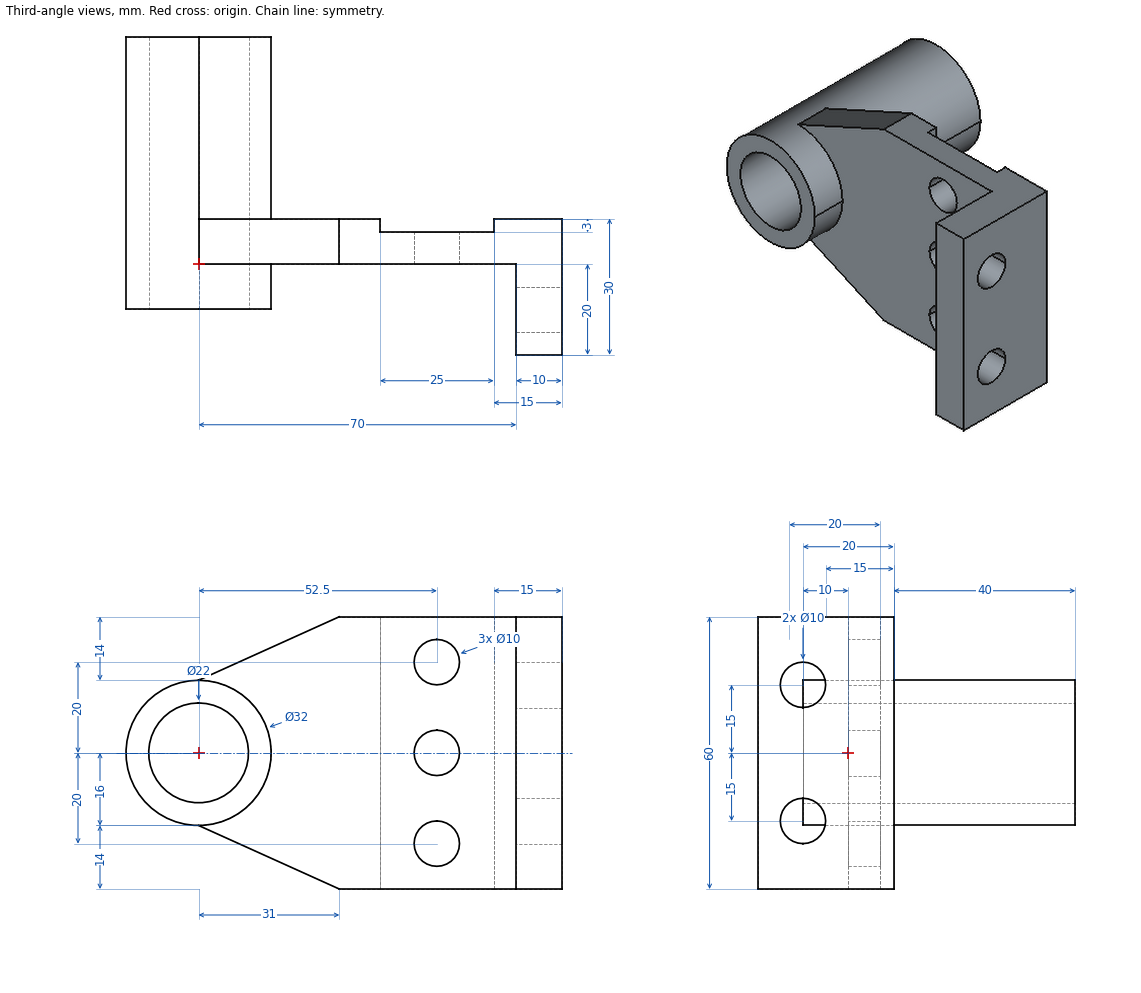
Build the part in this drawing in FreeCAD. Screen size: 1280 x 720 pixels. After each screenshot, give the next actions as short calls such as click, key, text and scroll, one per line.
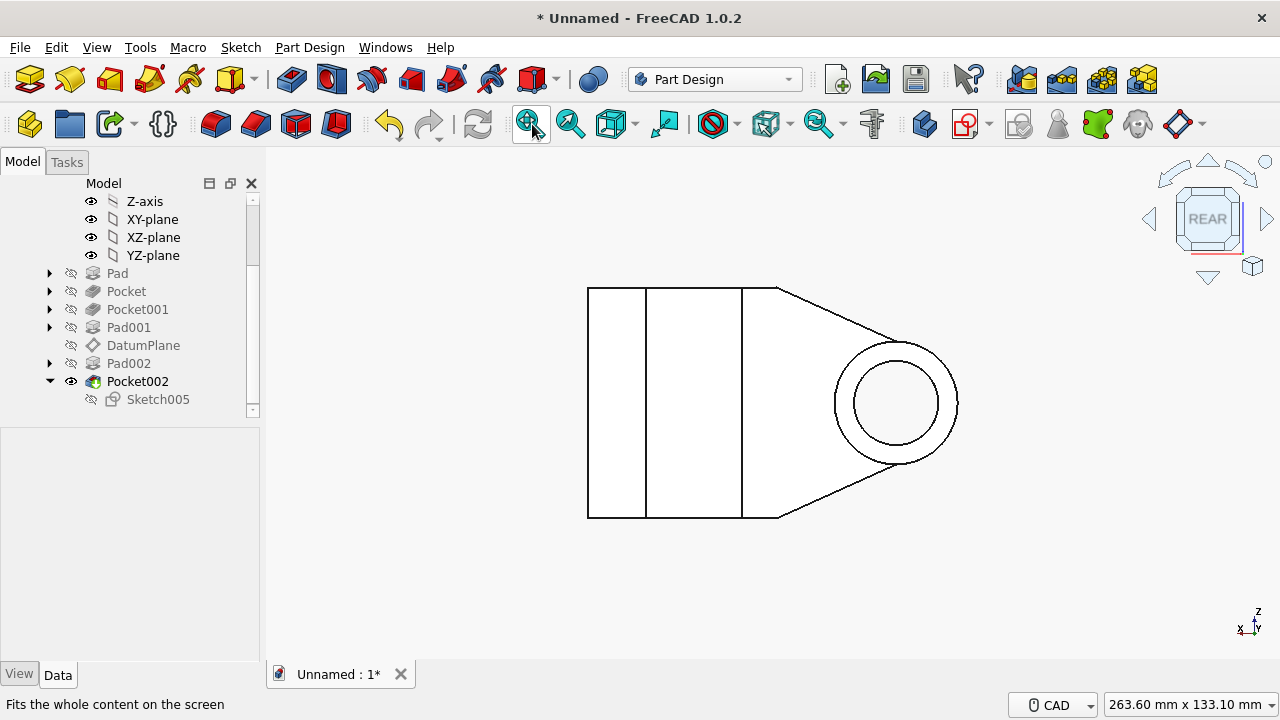
click(694, 336)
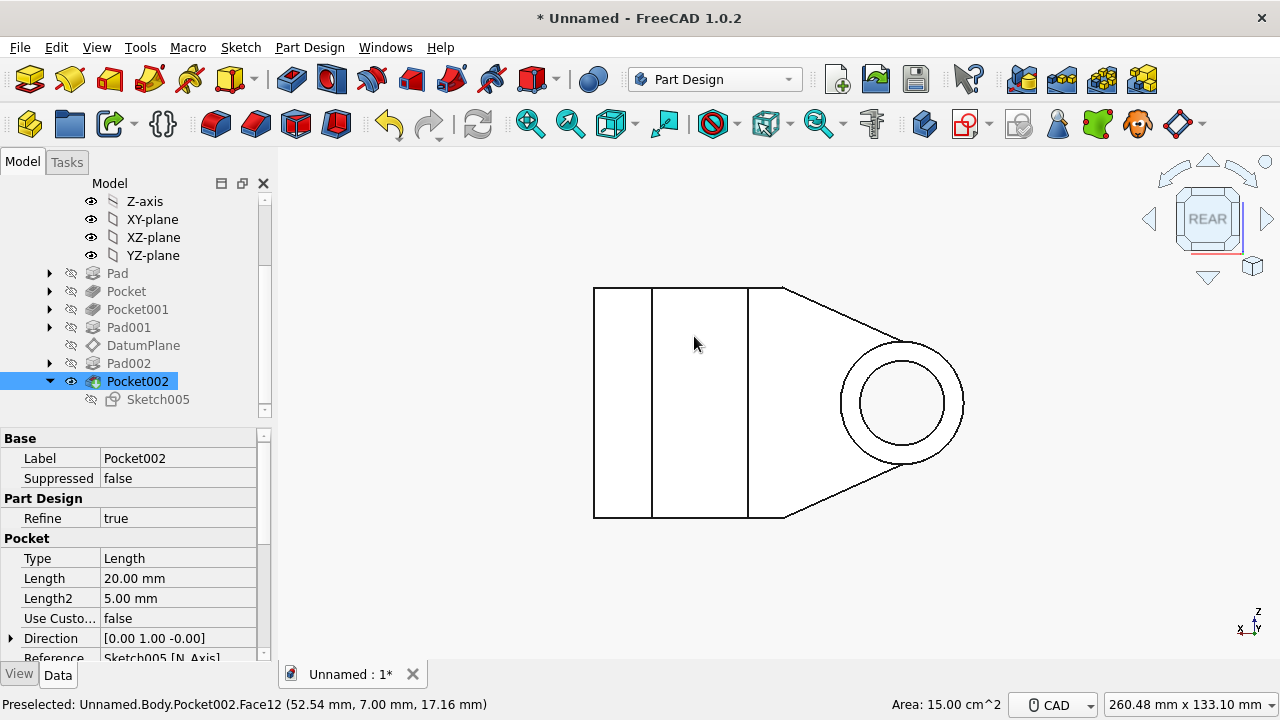
click(966, 124)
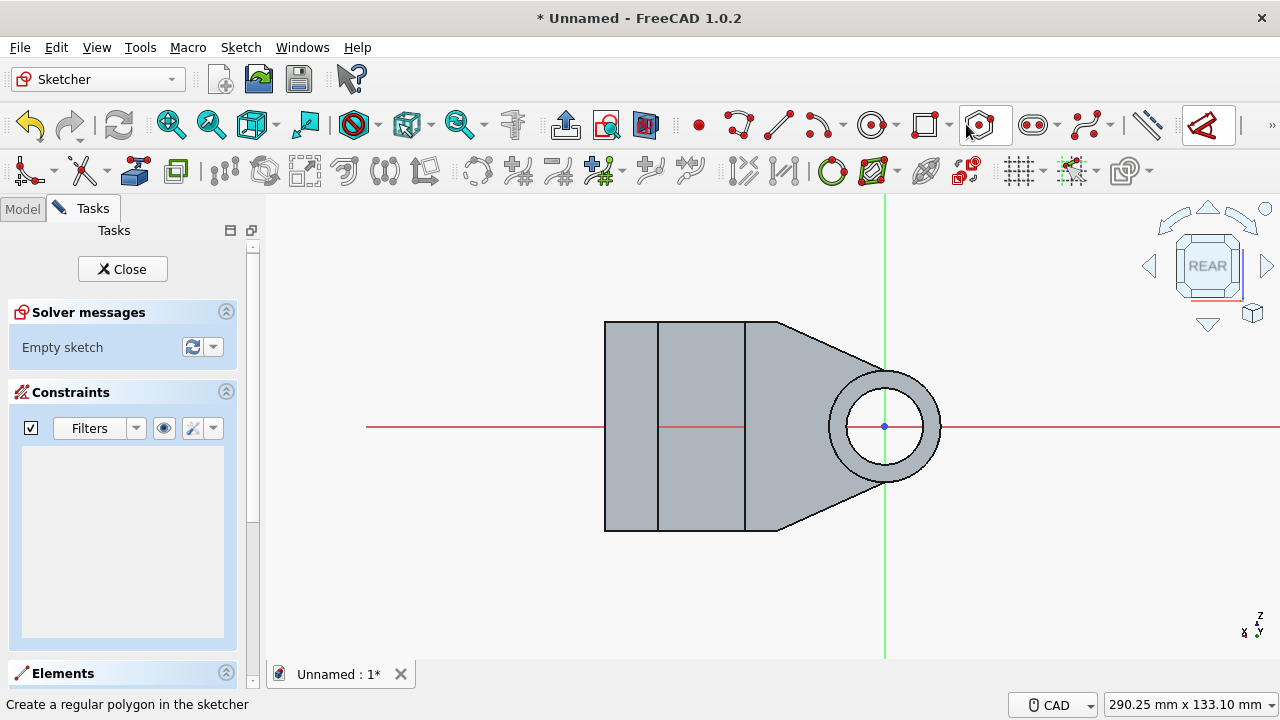
scroll(881, 426, up, 3)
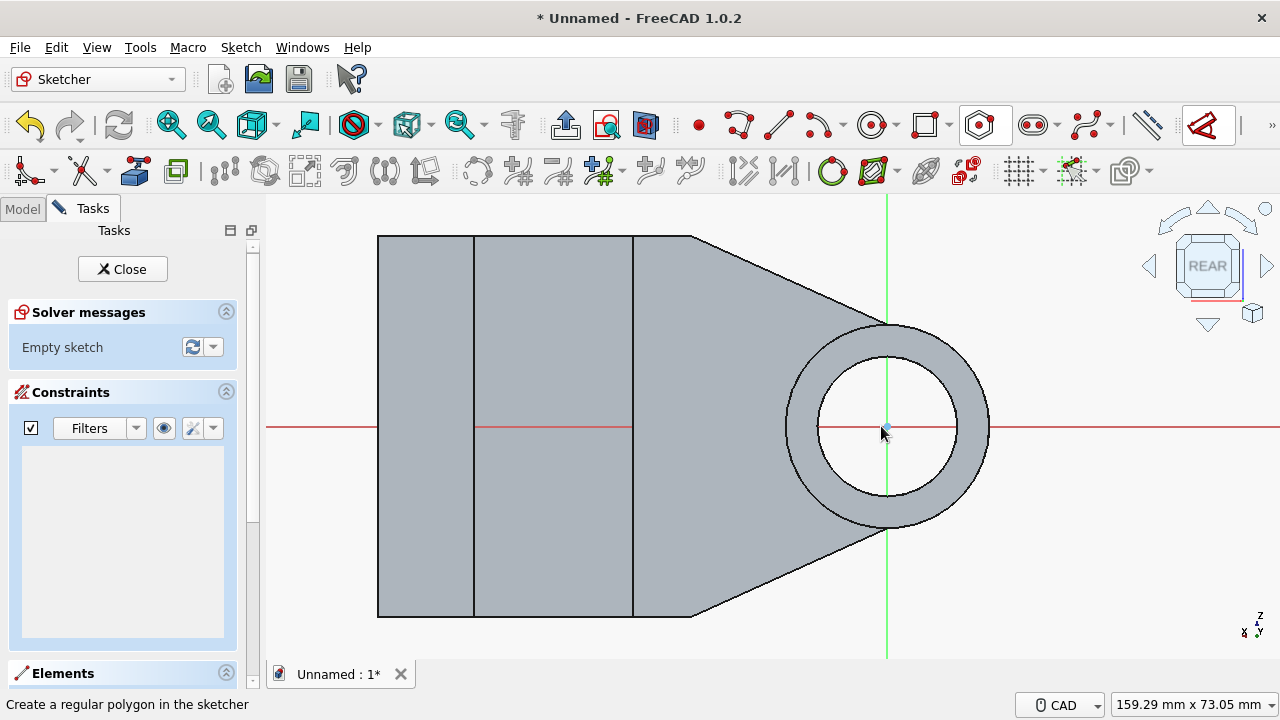
key(g)
key(c)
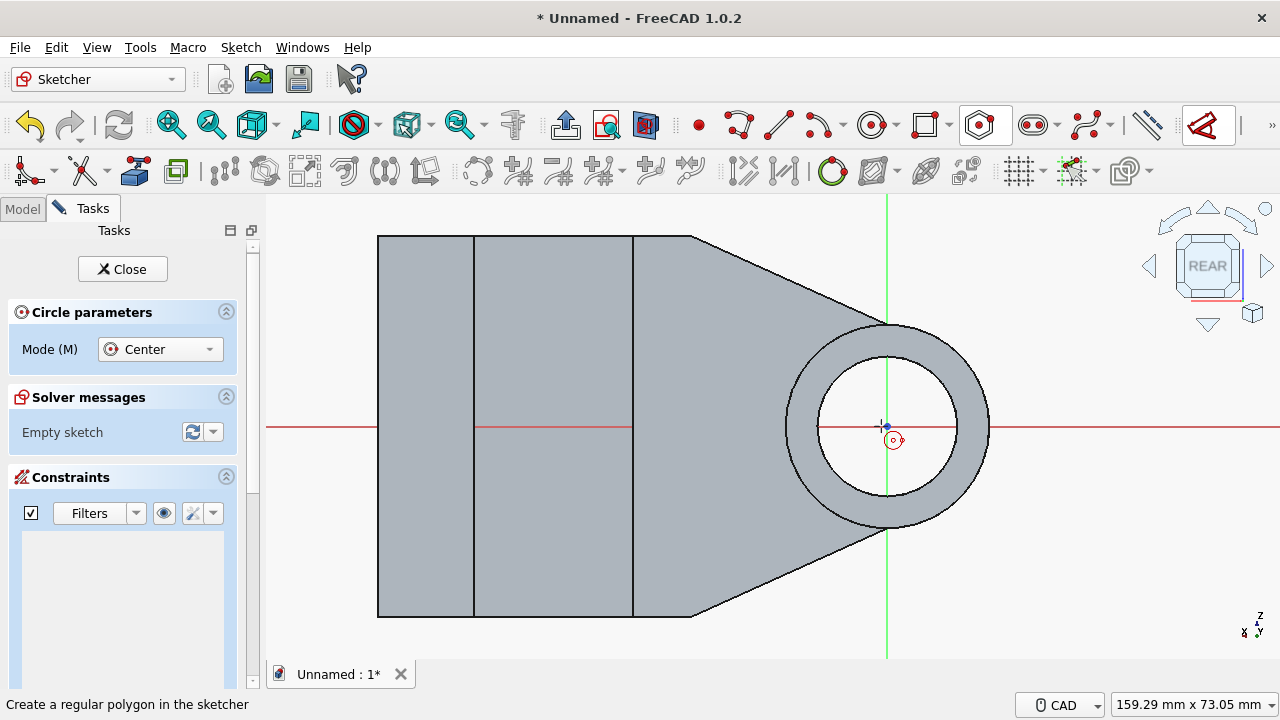
click(553, 299)
move(576, 277)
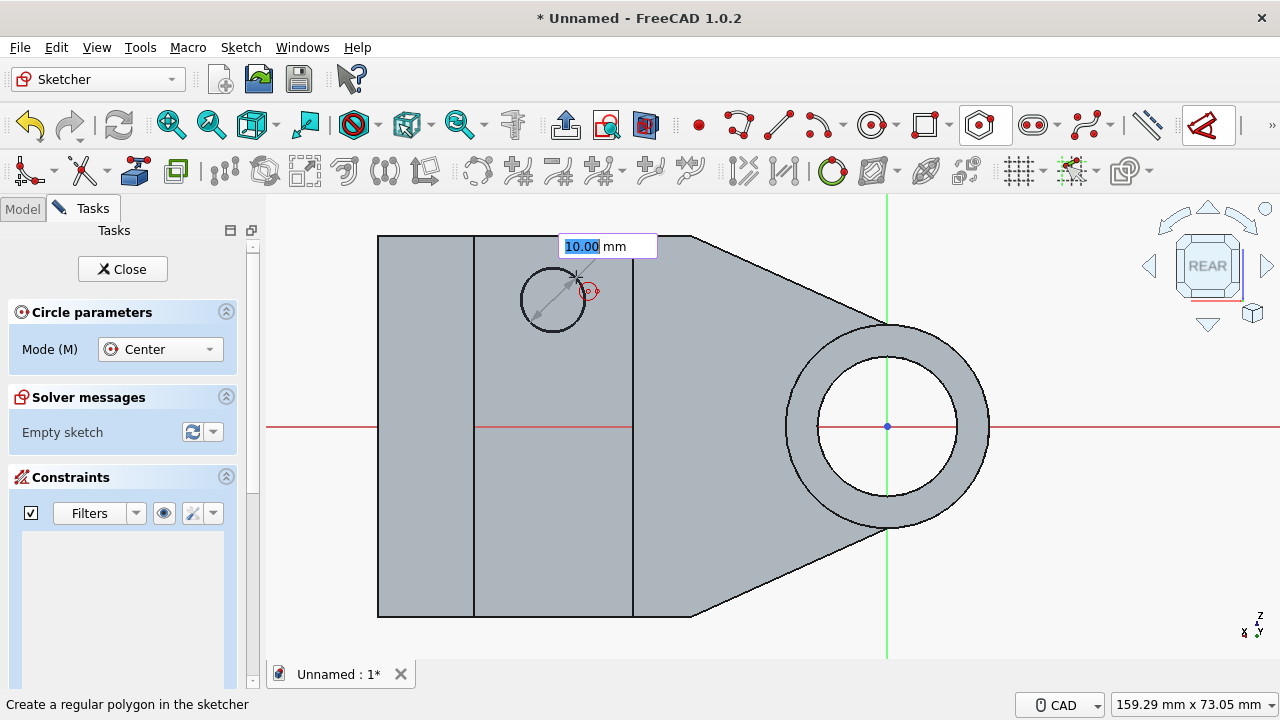
text(10)
key(Return)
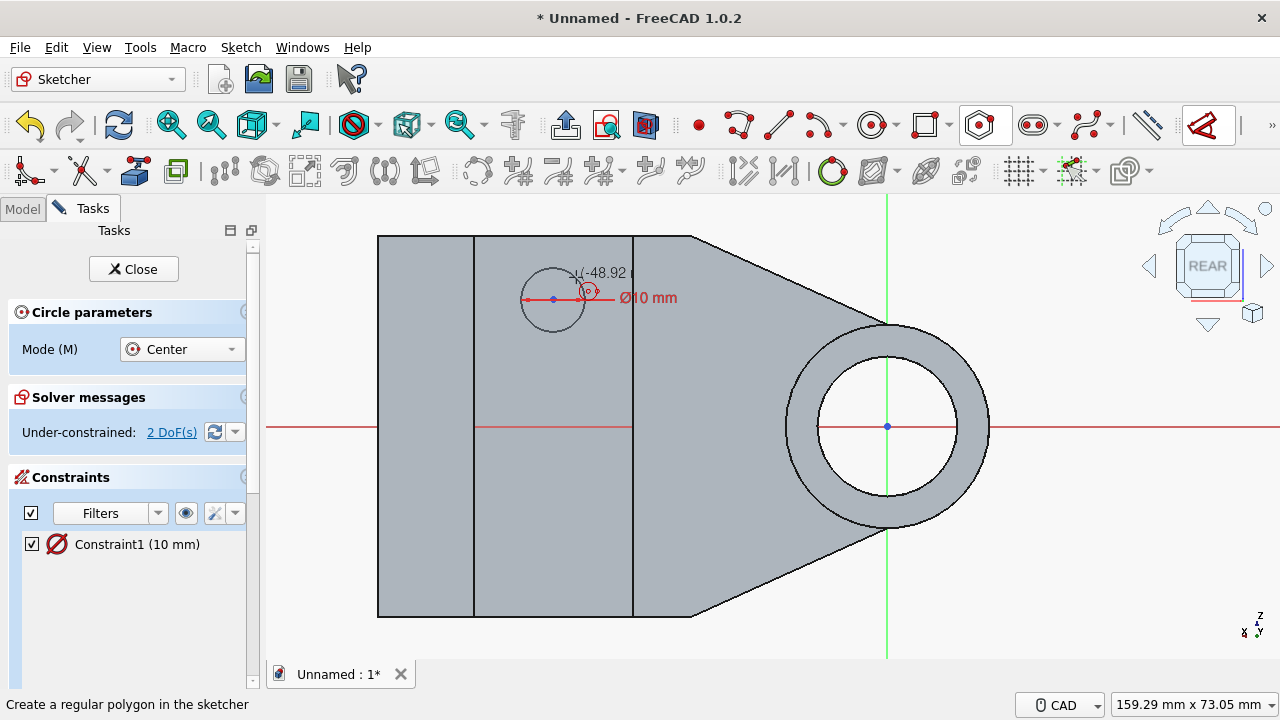
click(553, 426)
move(576, 404)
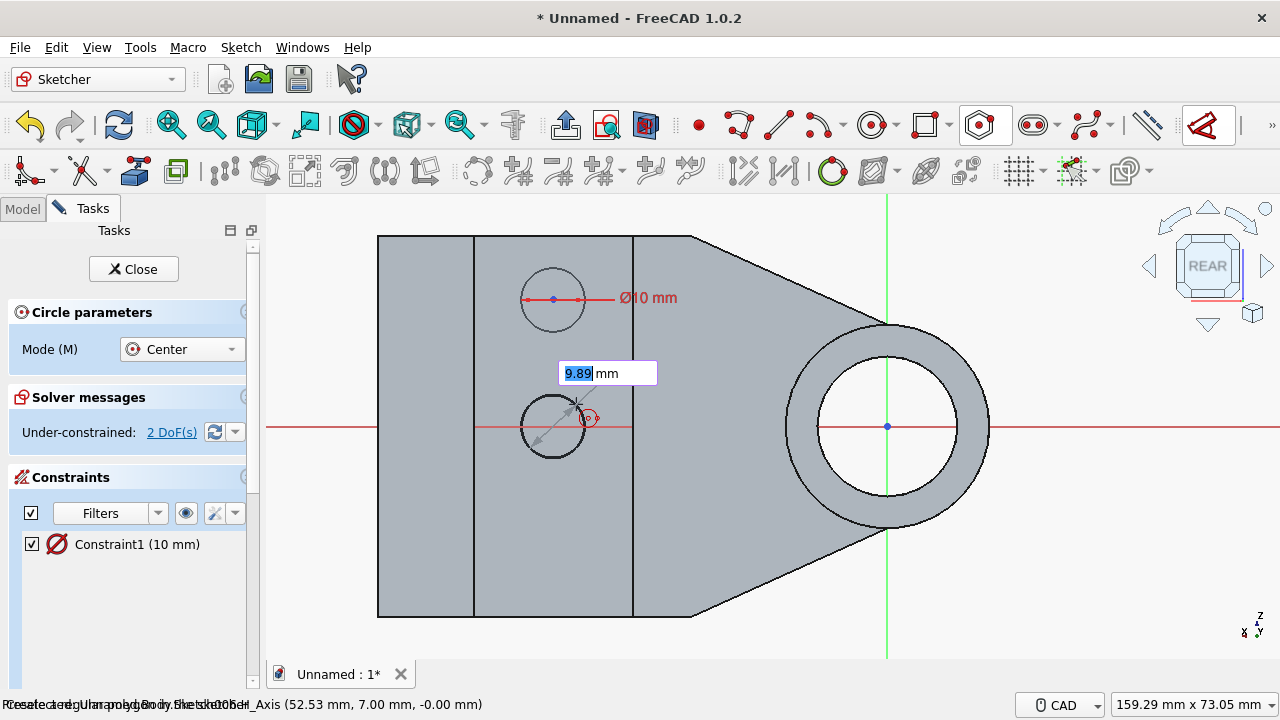
text(10)
key(Return)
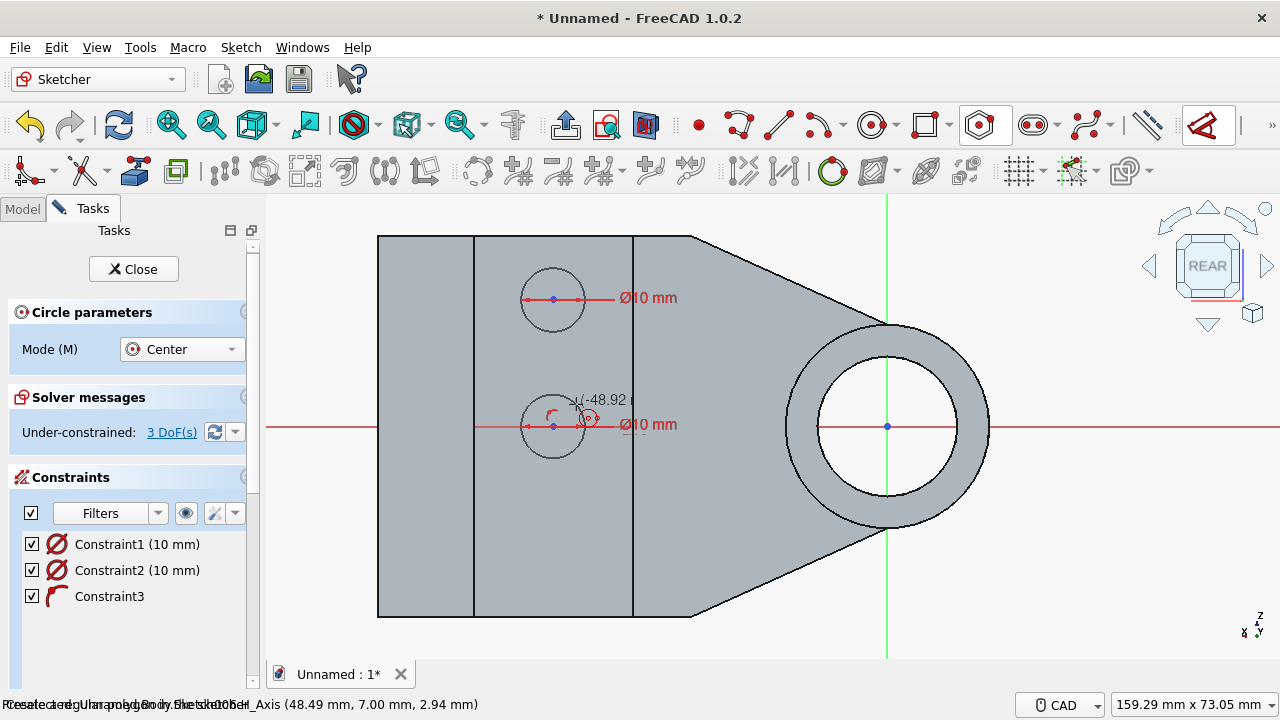
click(553, 554)
move(576, 531)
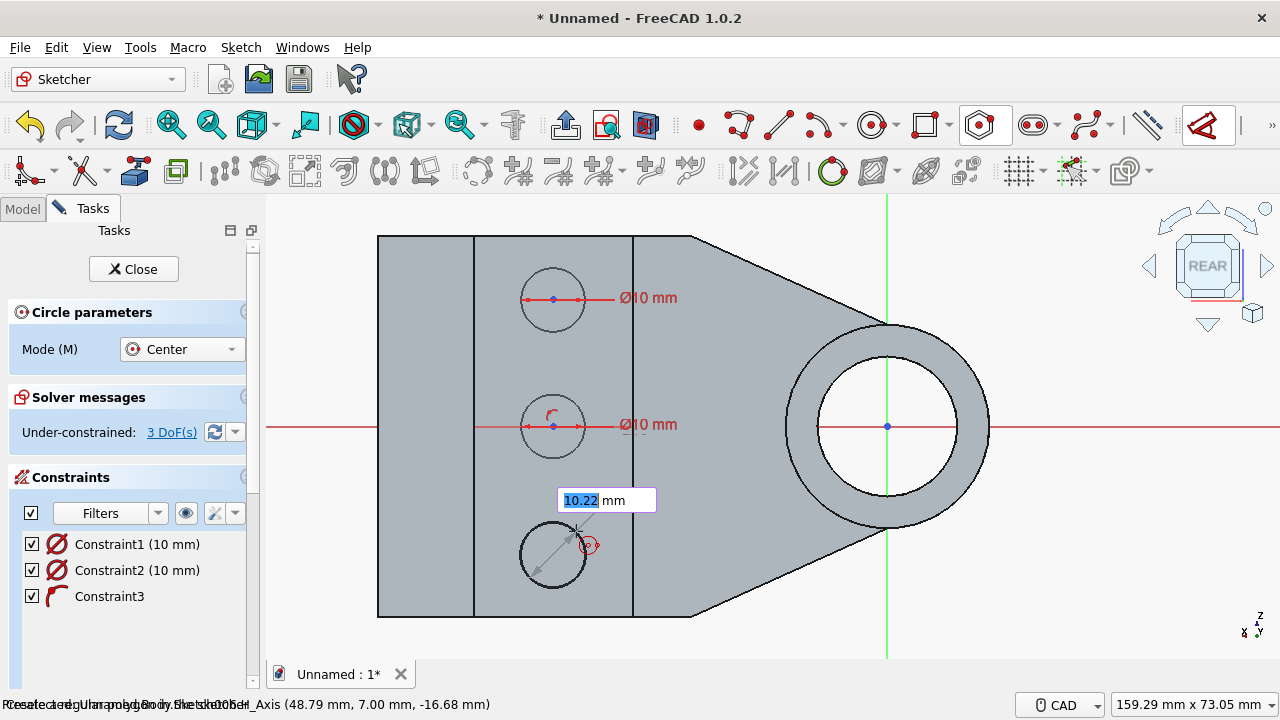
text(10)
key(Return)
key(Escape)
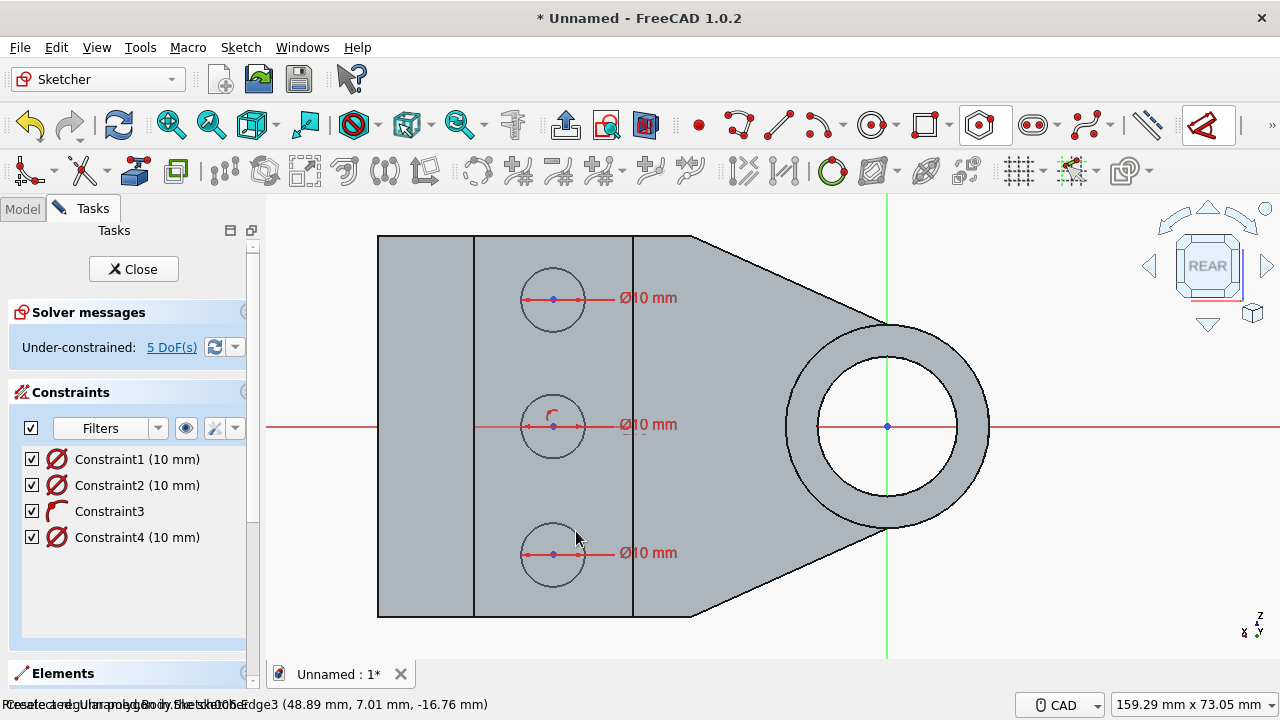
click(553, 300)